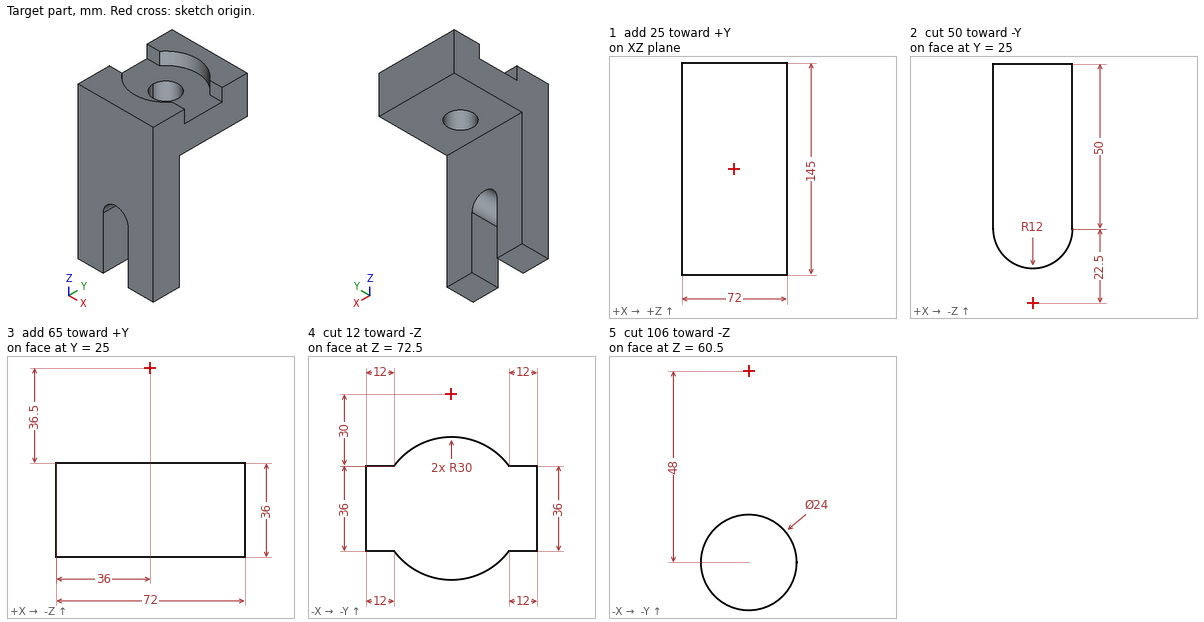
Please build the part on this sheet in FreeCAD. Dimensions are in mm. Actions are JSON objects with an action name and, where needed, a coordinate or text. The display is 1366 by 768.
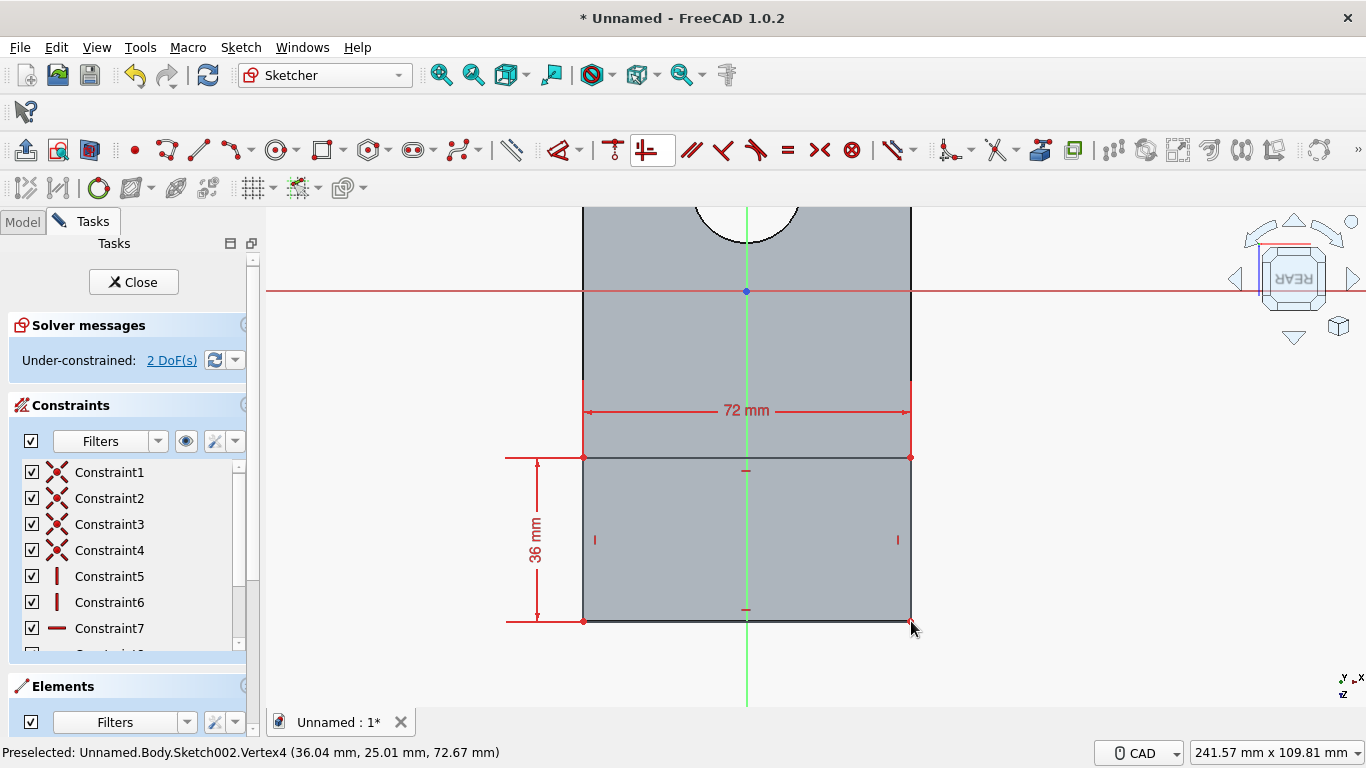
{"action": "left_click", "coordinate": [558, 150]}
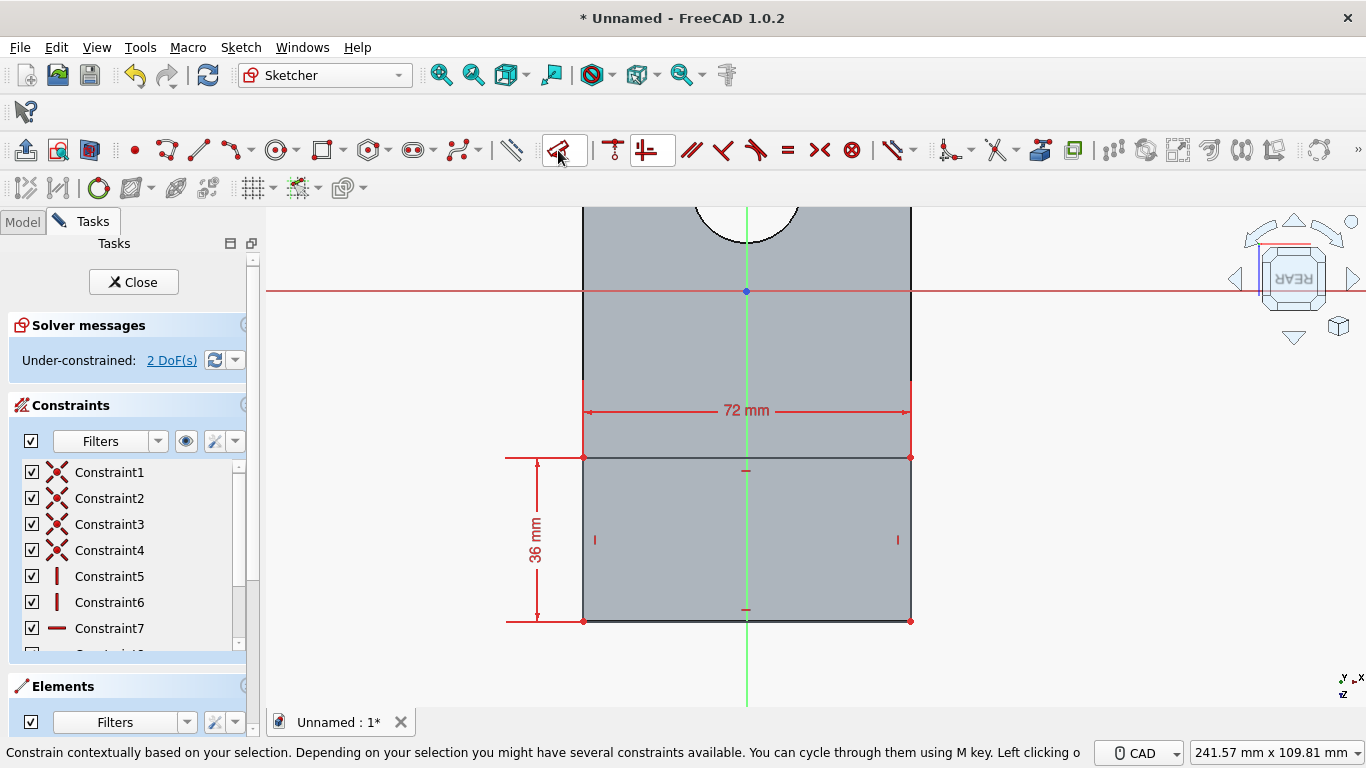
{"action": "left_click", "coordinate": [583, 458]}
{"action": "left_click", "coordinate": [665, 257]}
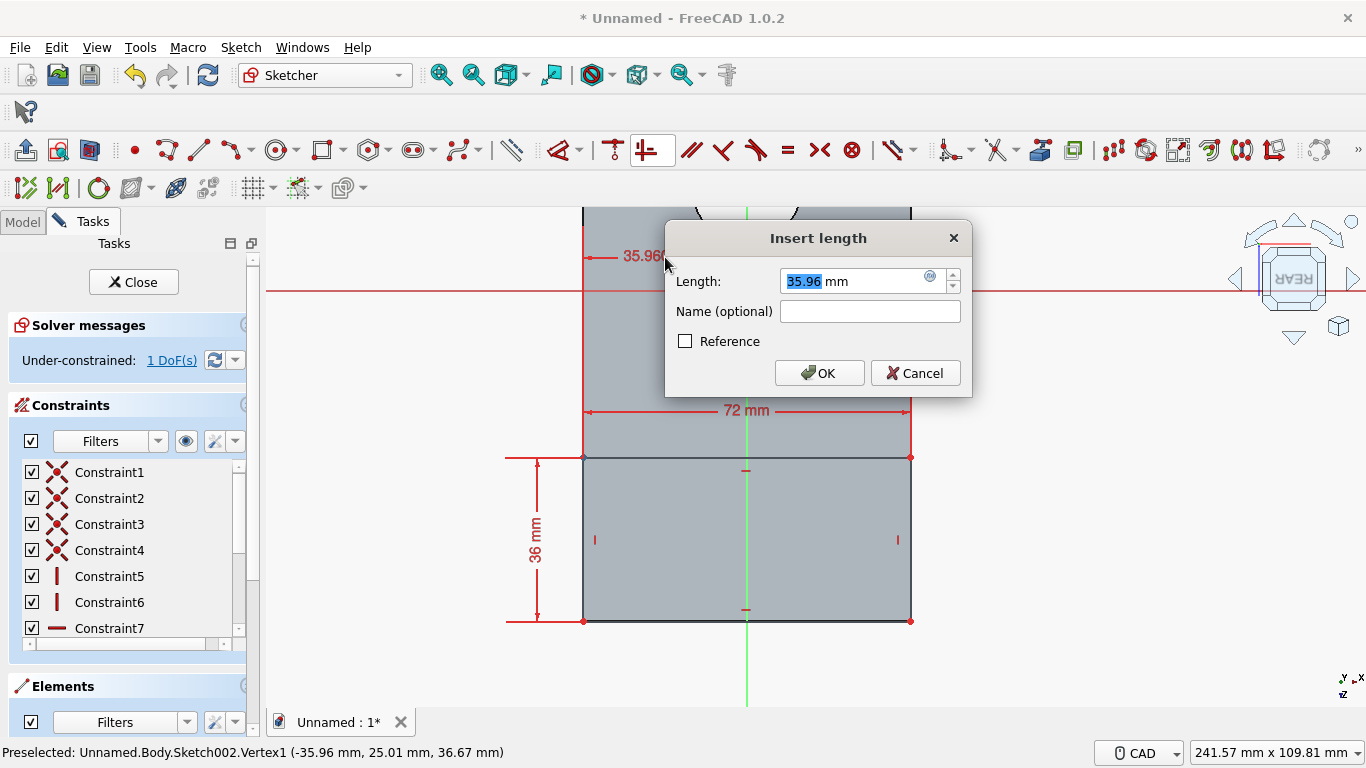
{"action": "type", "text": "36"}
{"action": "key", "text": "Return"}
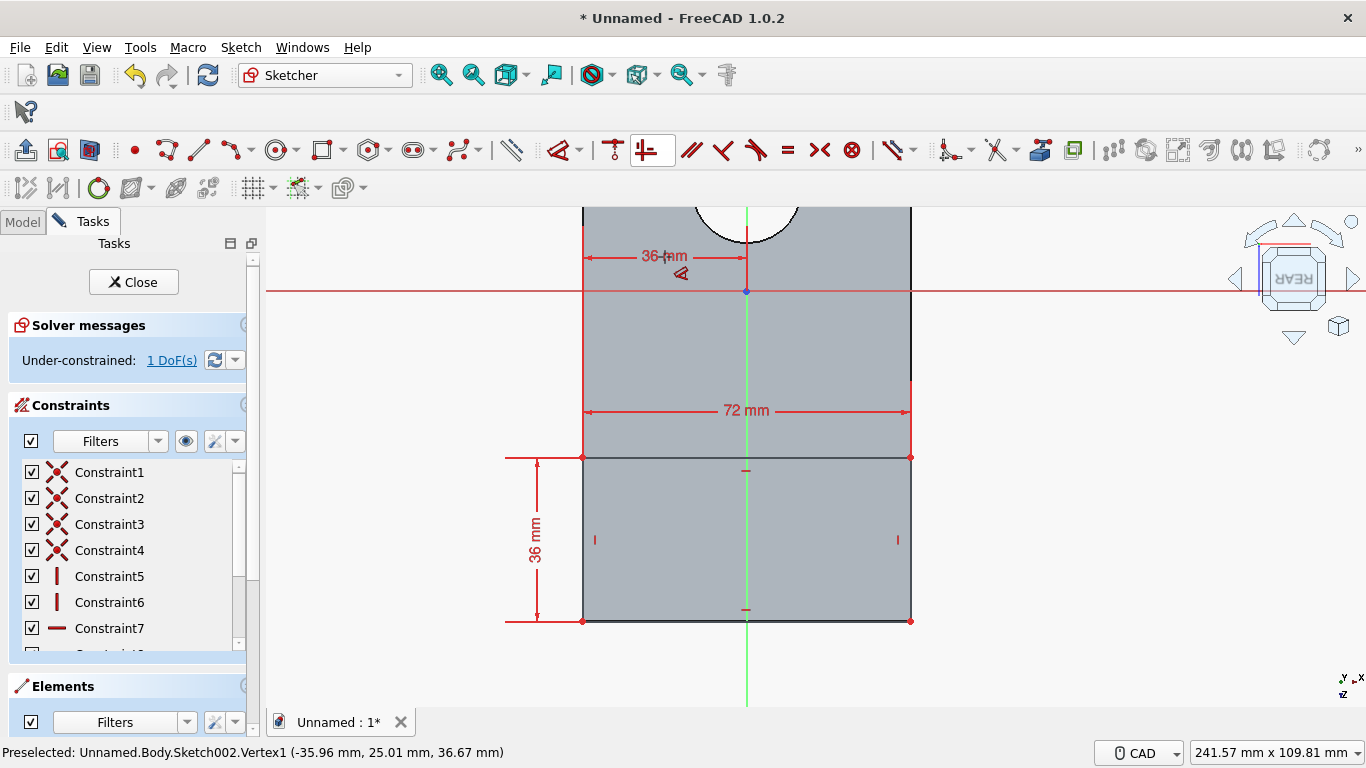
{"action": "left_click", "coordinate": [583, 458]}
{"action": "left_click", "coordinate": [549, 375]}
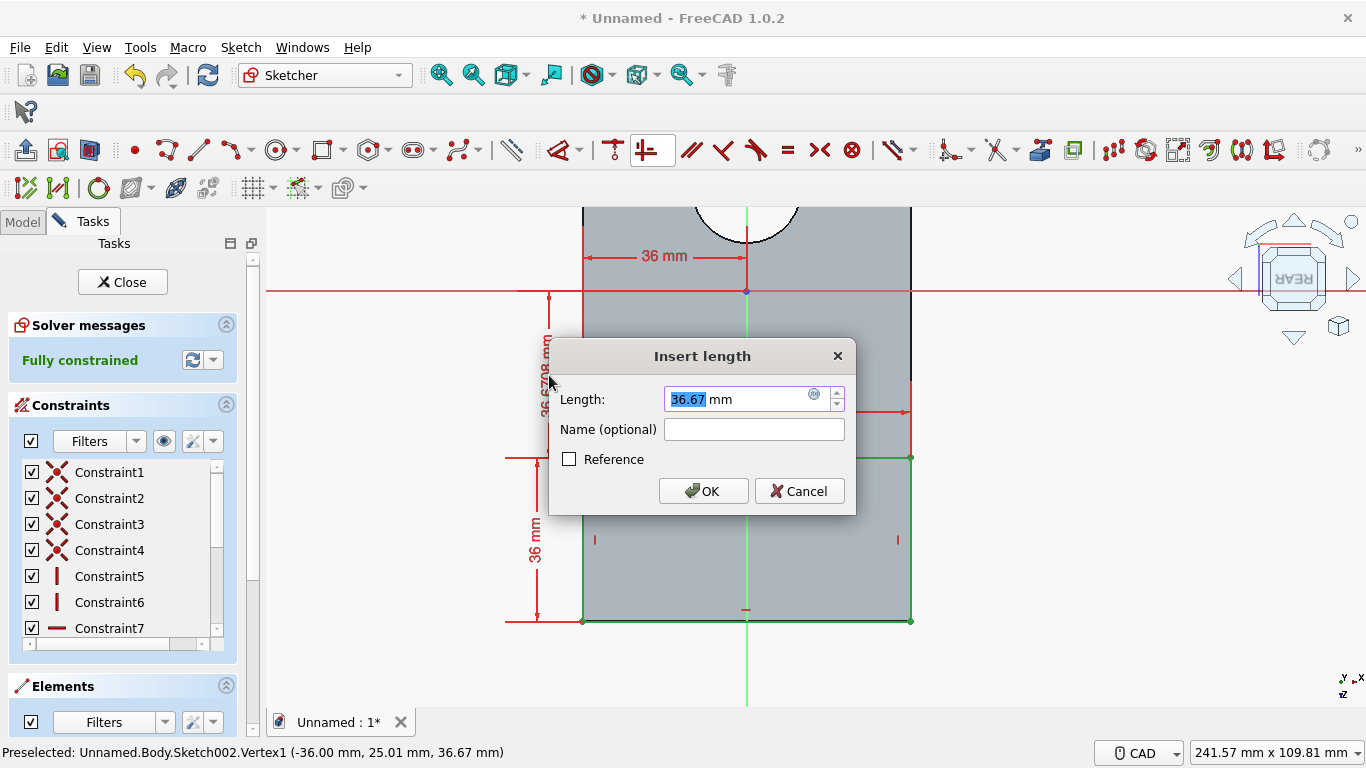
{"action": "type", "text": "36.5"}
{"action": "key", "text": "Return"}
{"action": "key", "text": "Escape"}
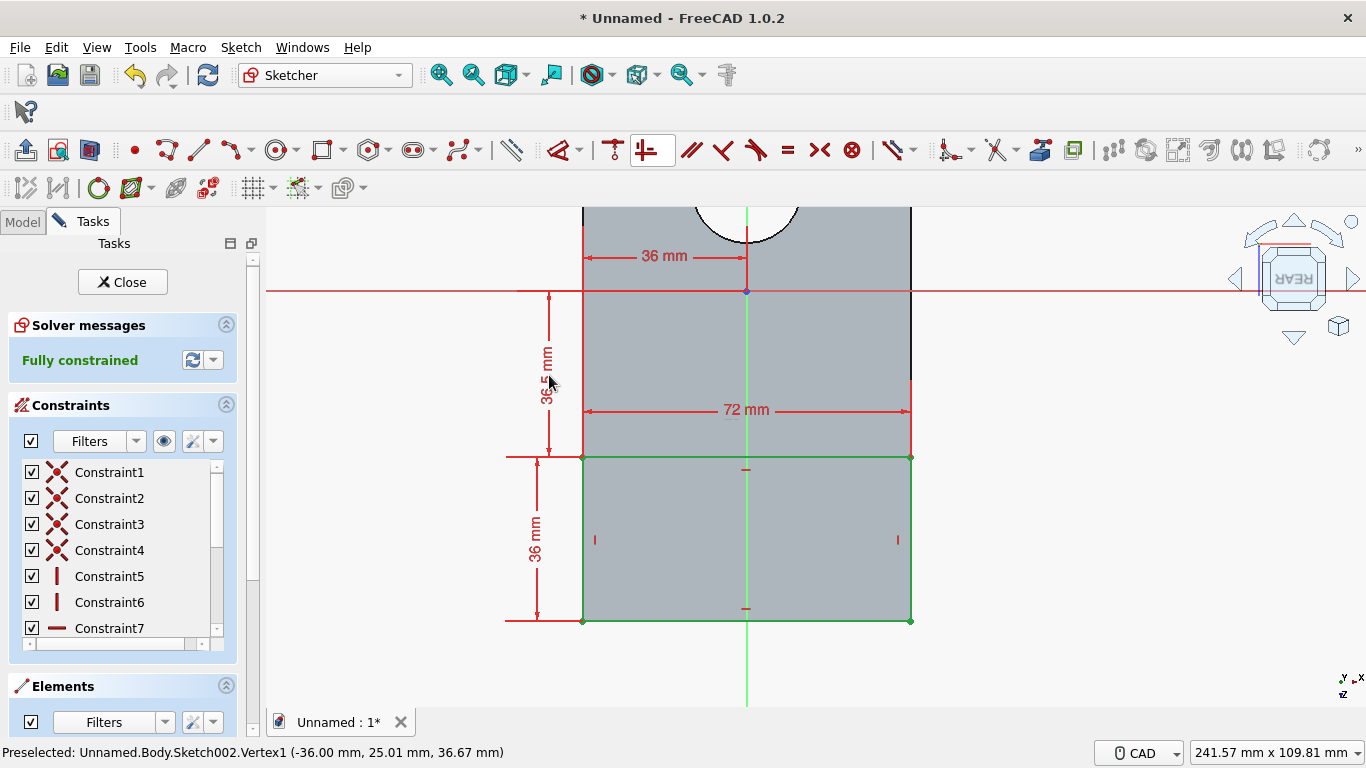
{"action": "left_click", "coordinate": [123, 282]}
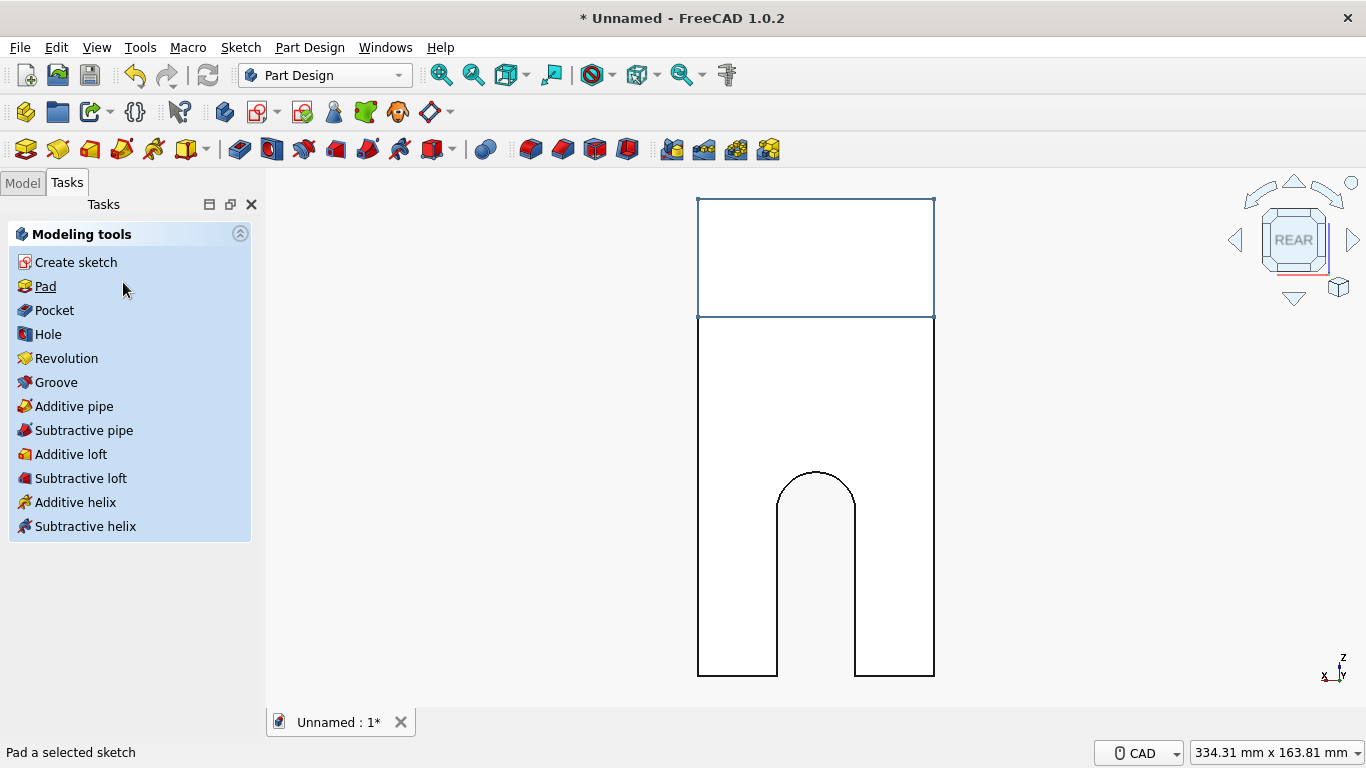
{"action": "left_click", "coordinate": [26, 150]}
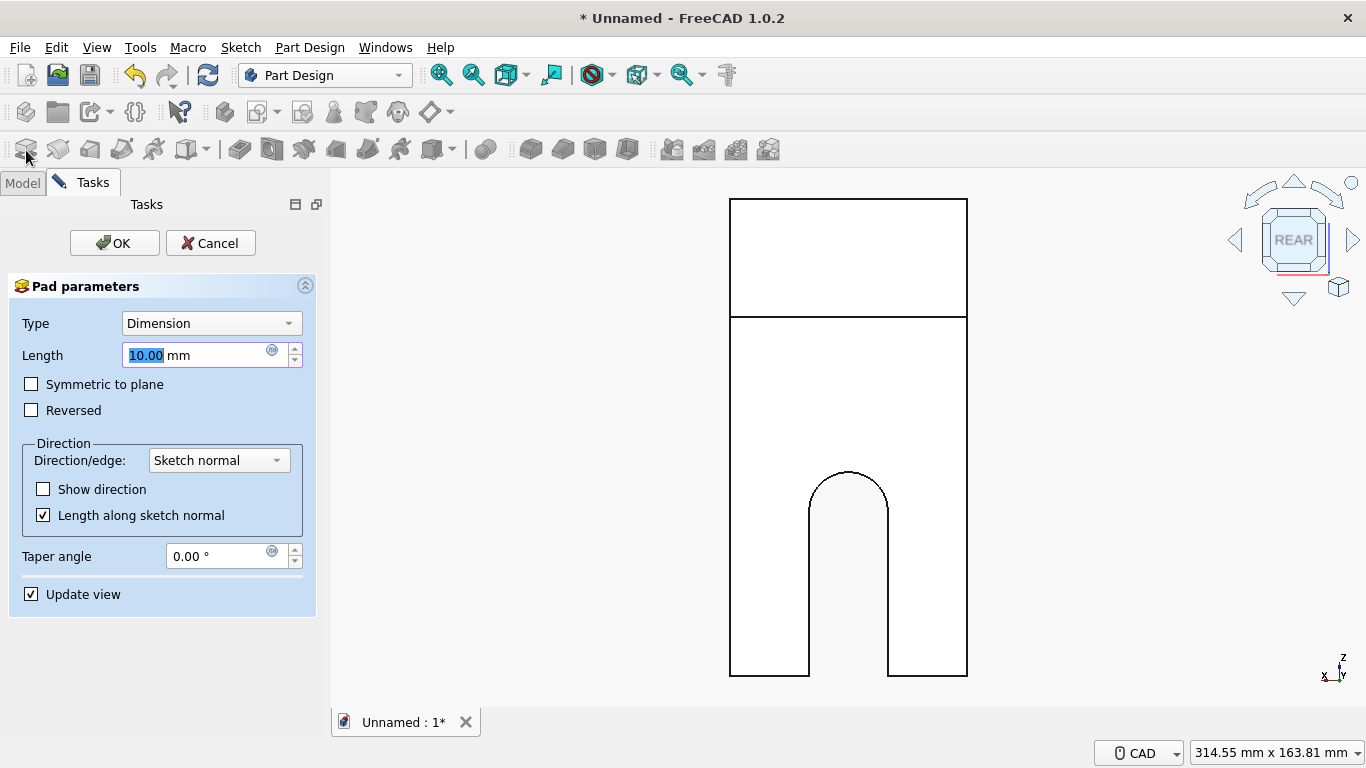
{"action": "type", "text": "65"}
{"action": "key", "text": "Tab"}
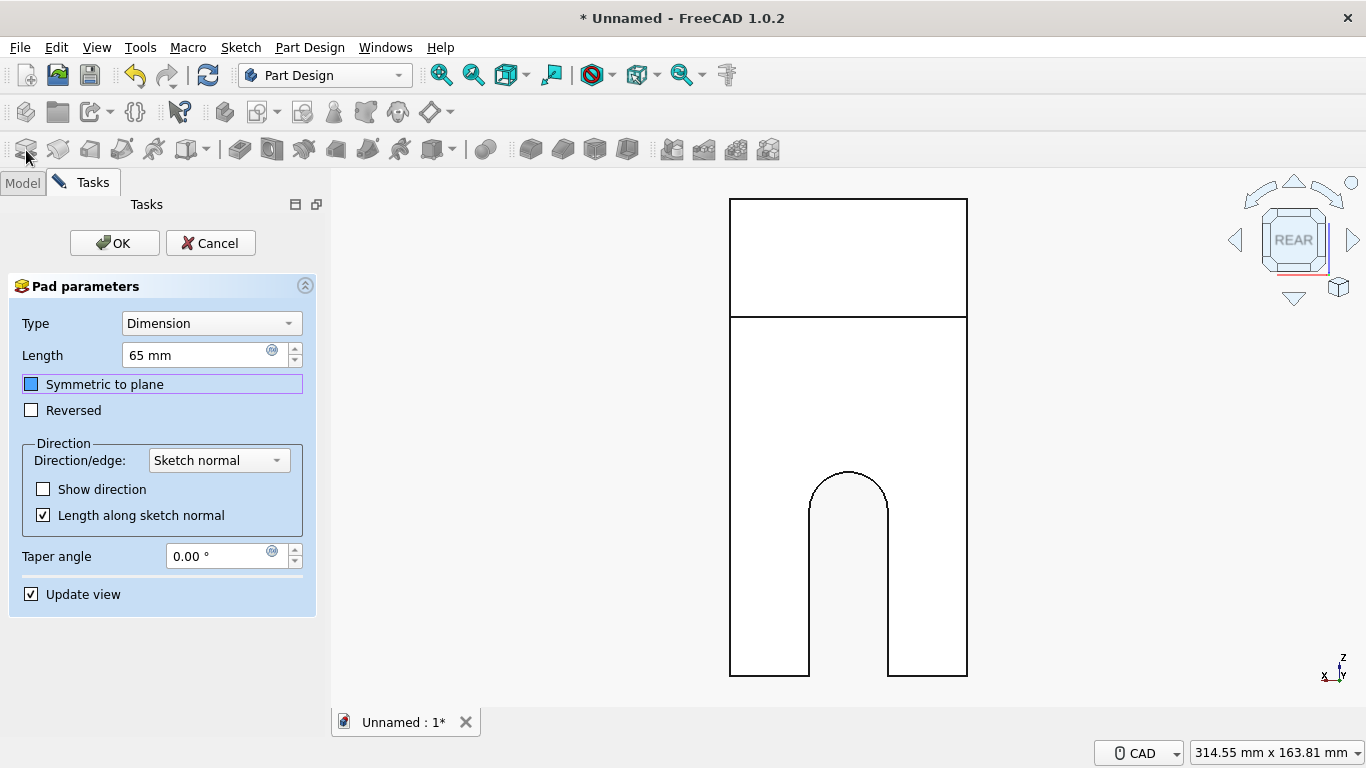
{"action": "left_click", "coordinate": [115, 243]}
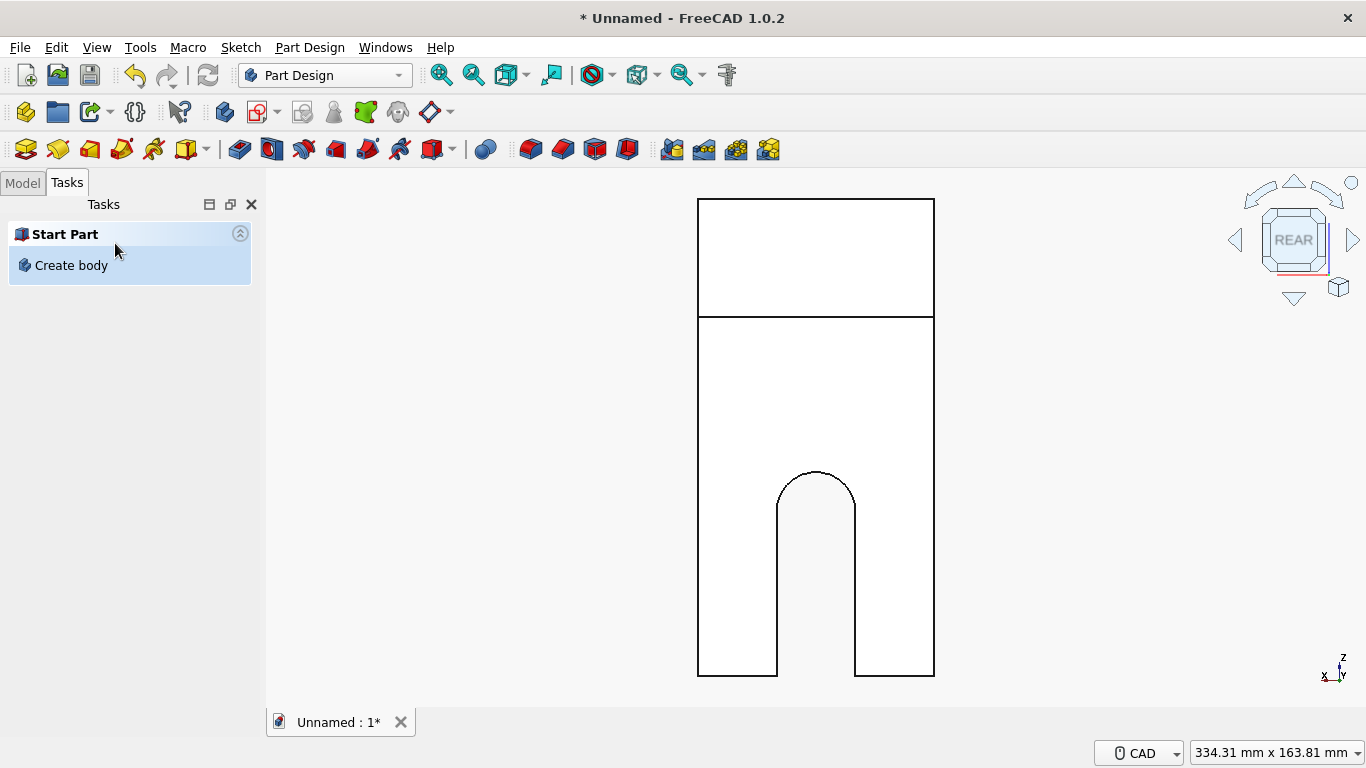
{"action": "key", "text": "0"}